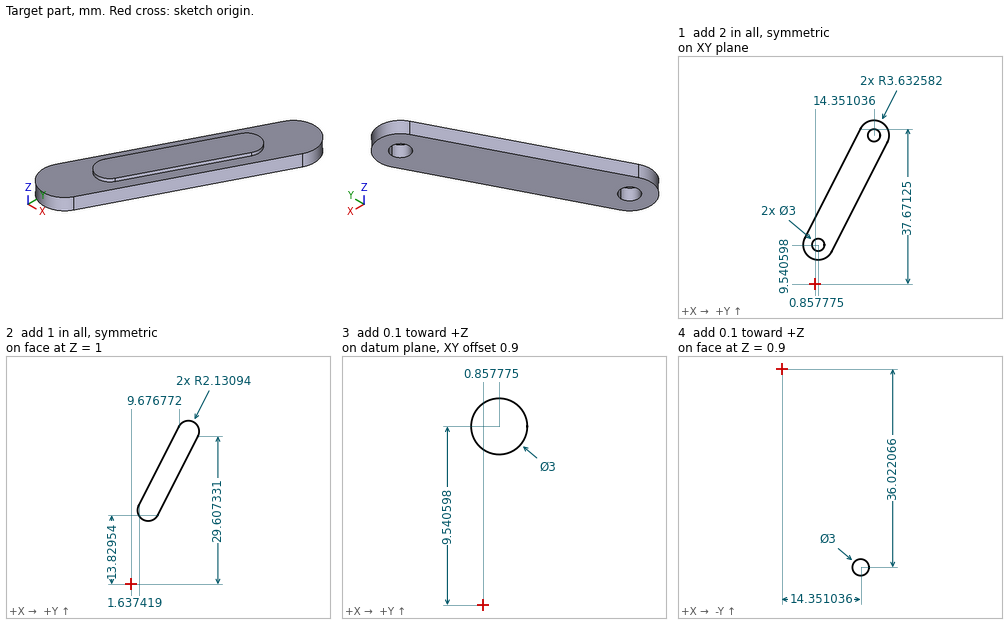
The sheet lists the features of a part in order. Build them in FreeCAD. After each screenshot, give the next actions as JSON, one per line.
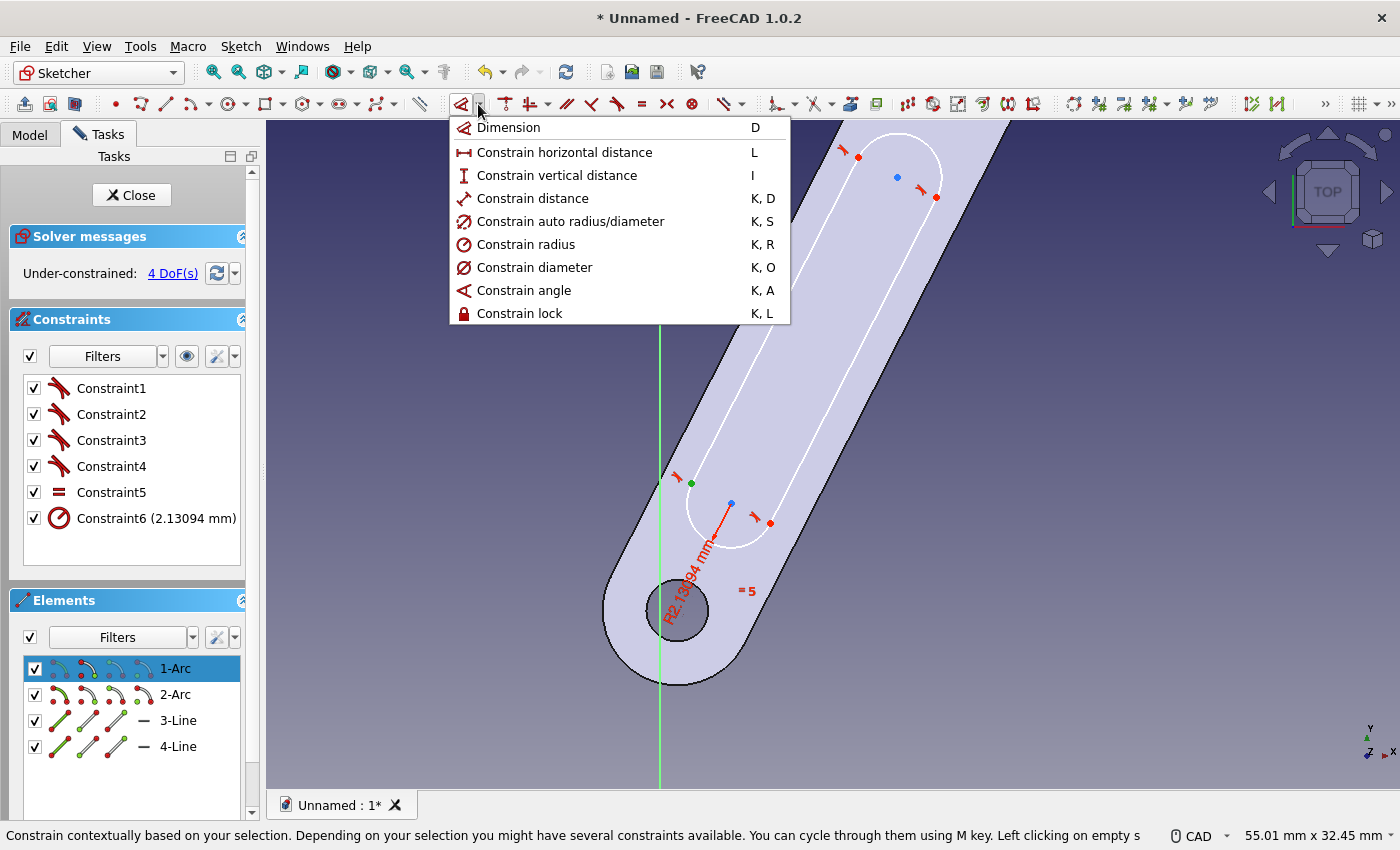
{"action": "left_click", "coordinate": [620, 152]}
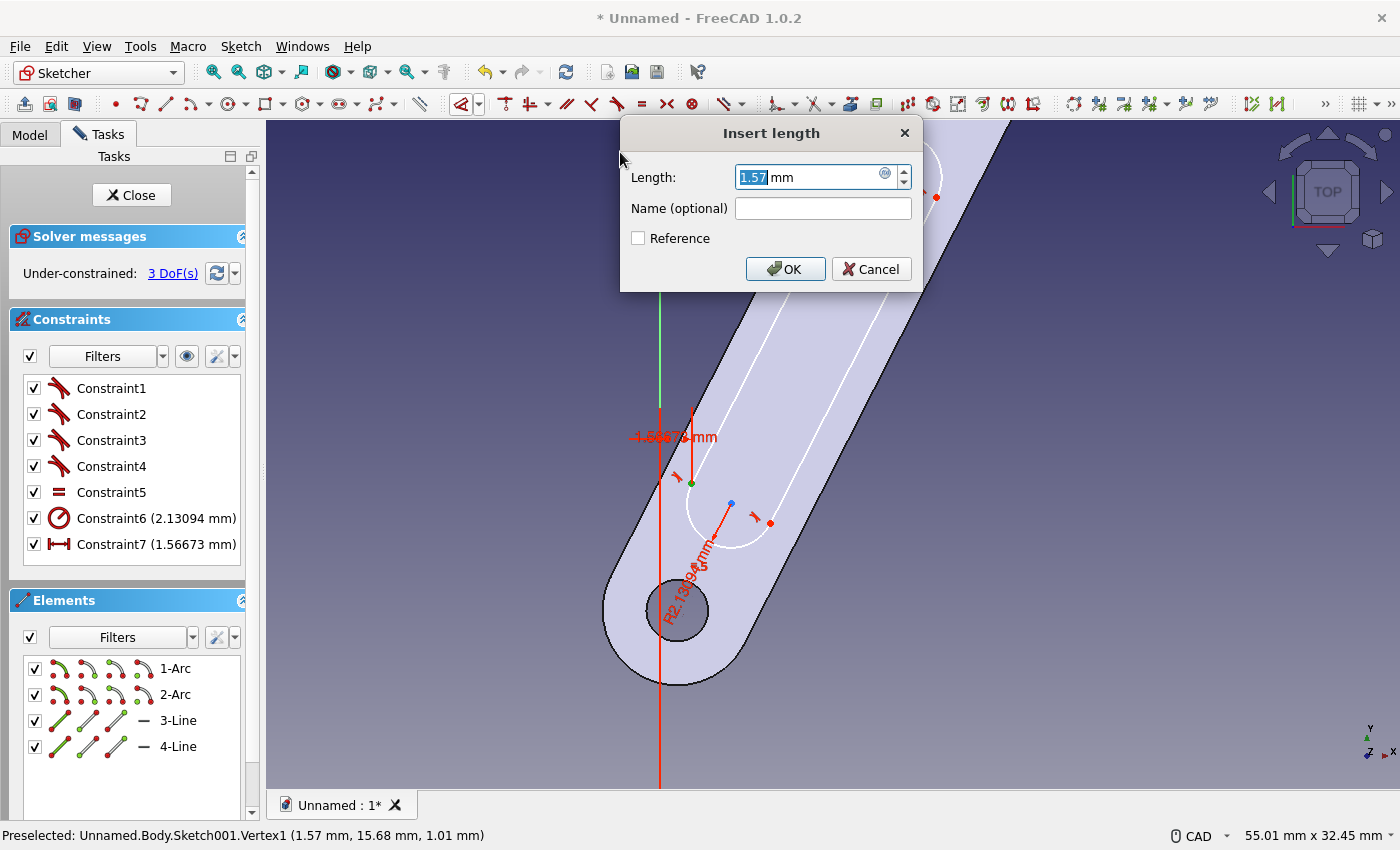
{"action": "type", "text": "1.637419"}
{"action": "key", "text": "Return"}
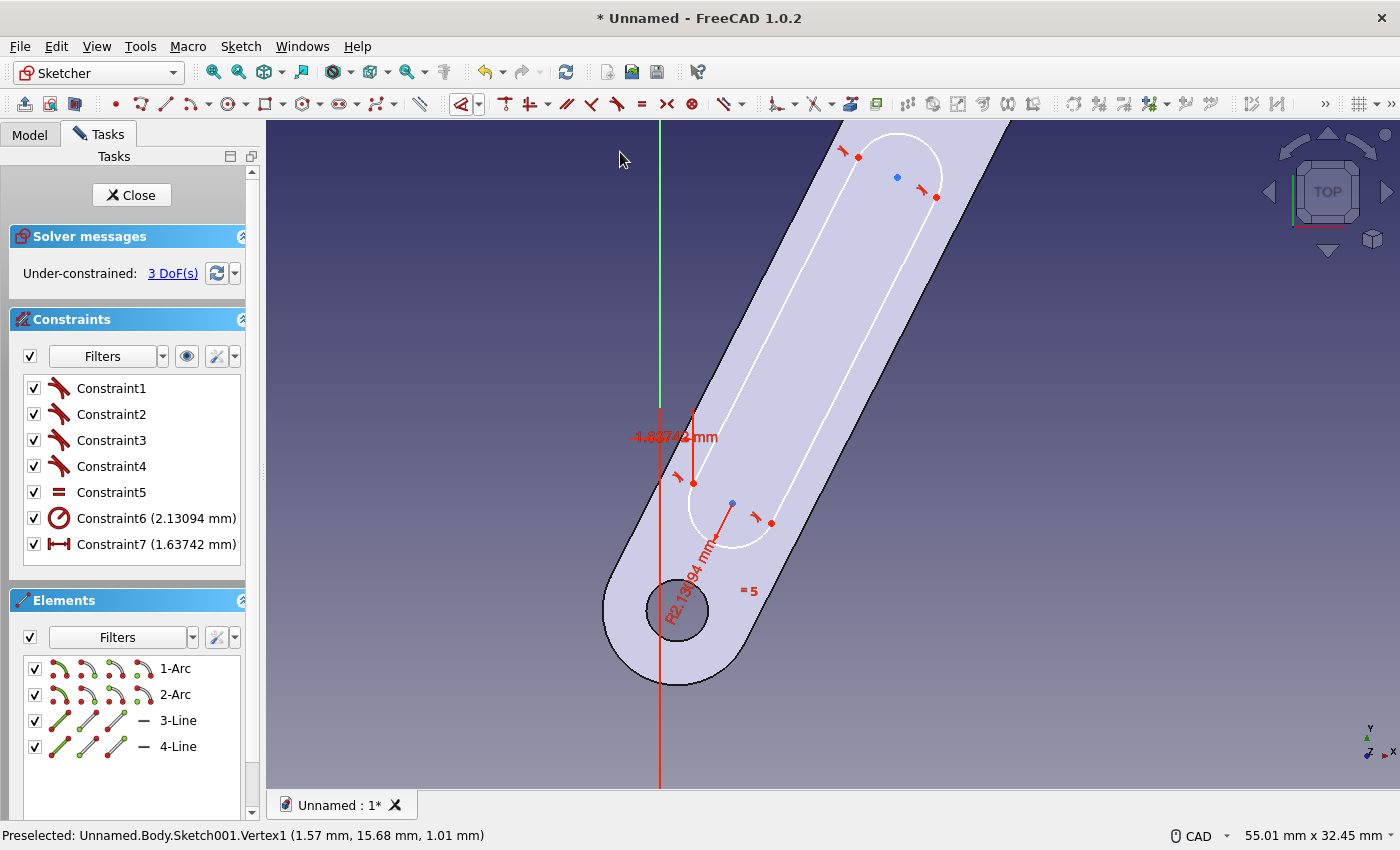
{"action": "left_click", "coordinate": [772, 524]}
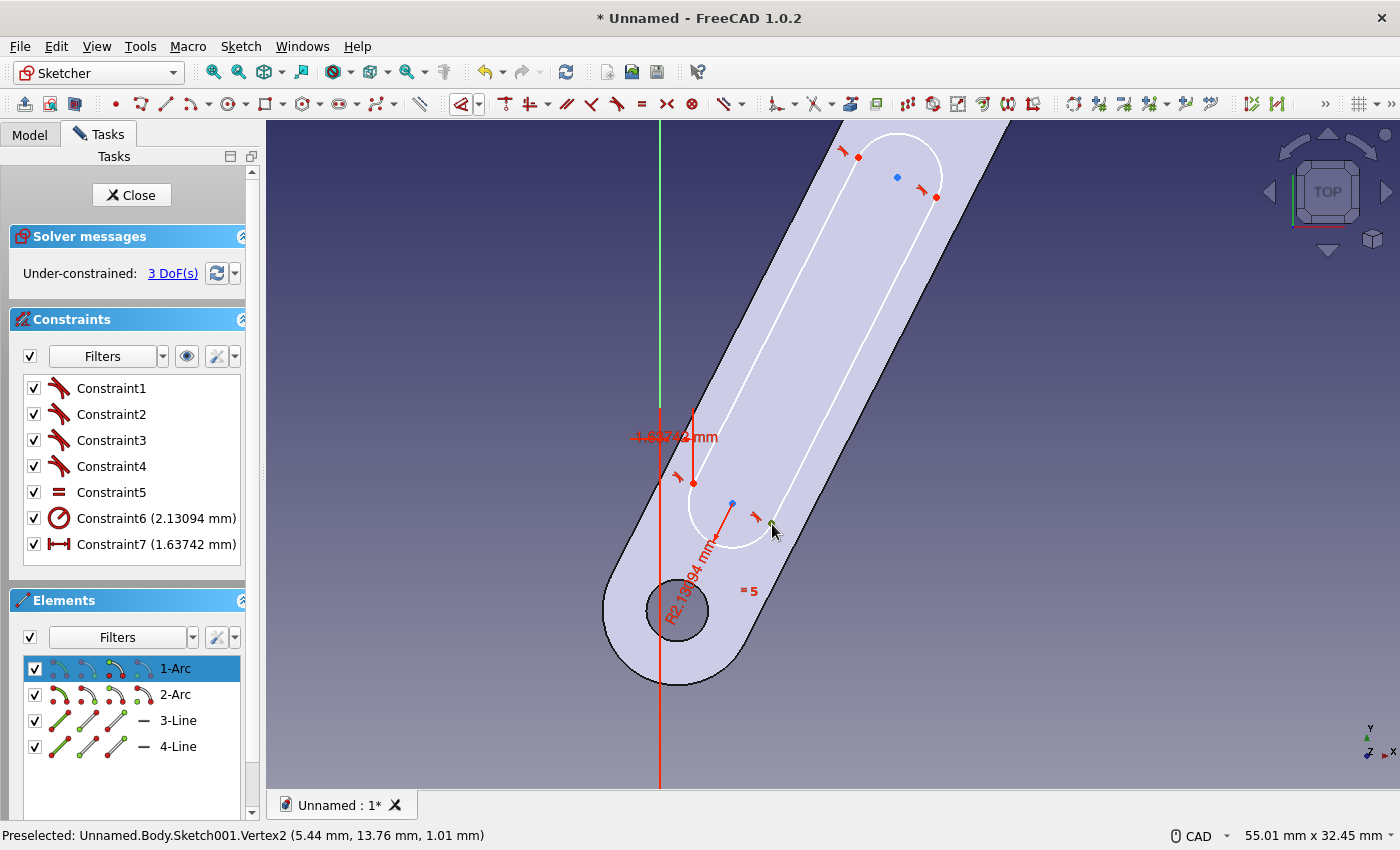
{"action": "key", "text": "i"}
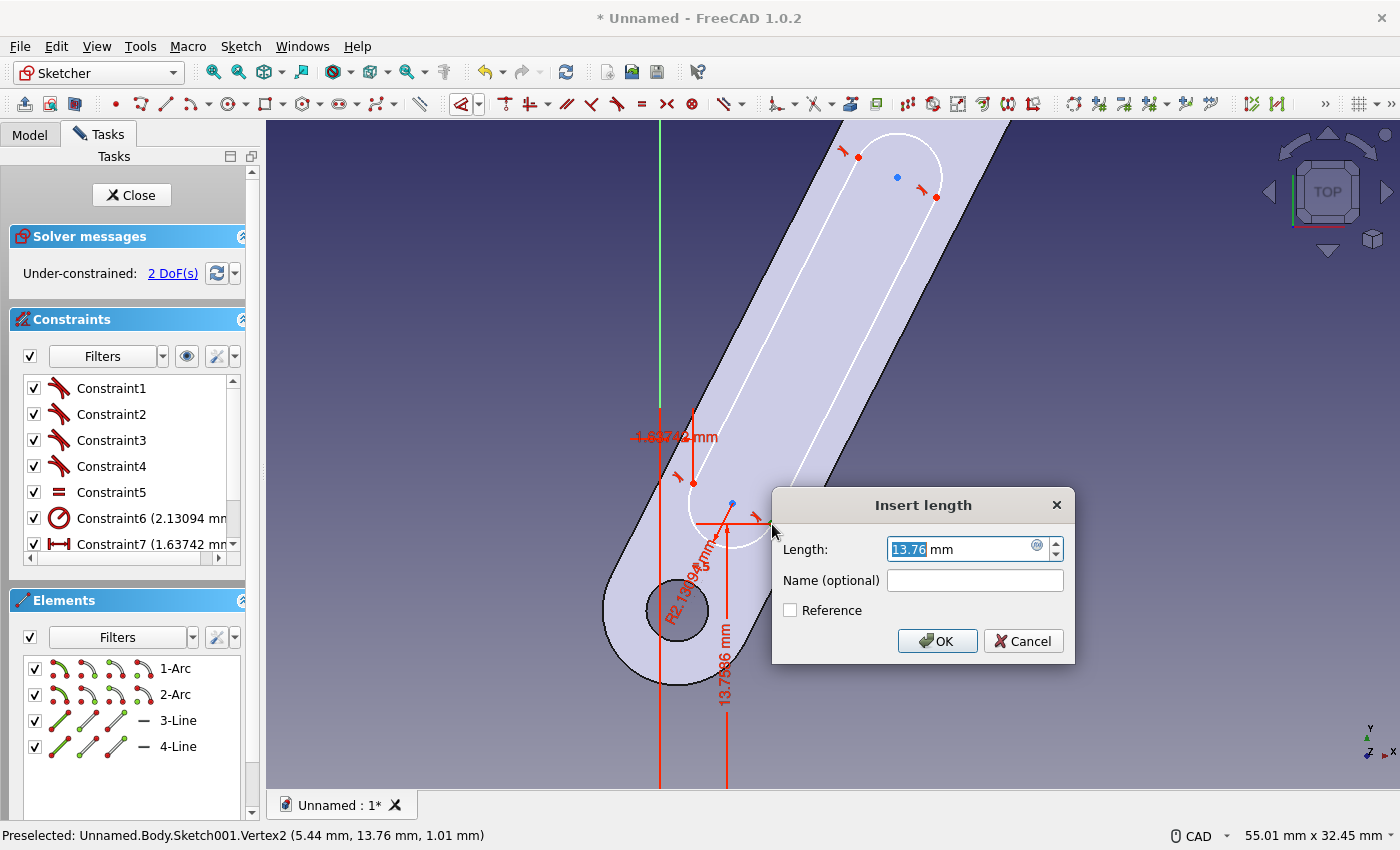
{"action": "type", "text": "13.82954"}
{"action": "key", "text": "Return"}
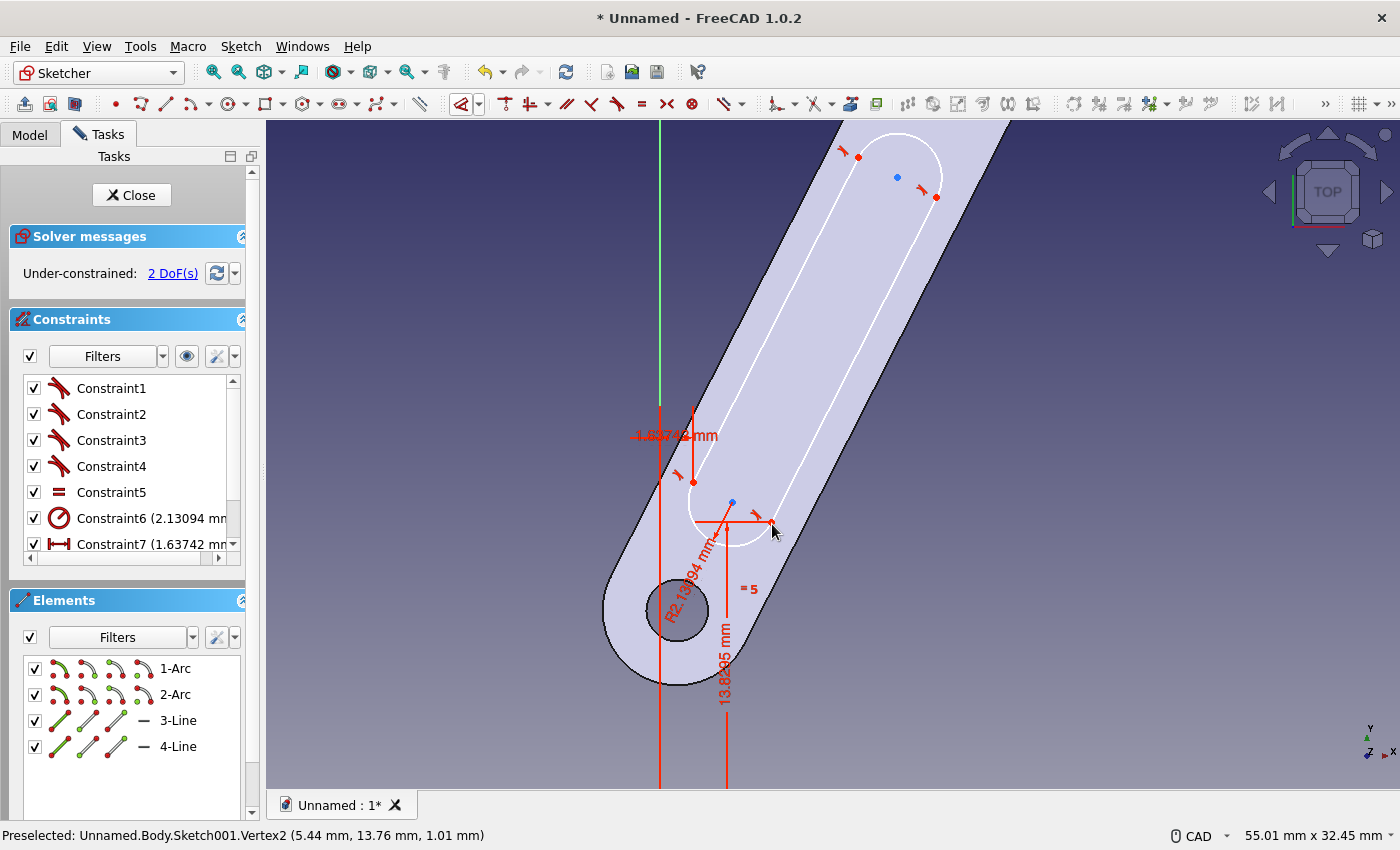
{"action": "left_click", "coordinate": [859, 158]}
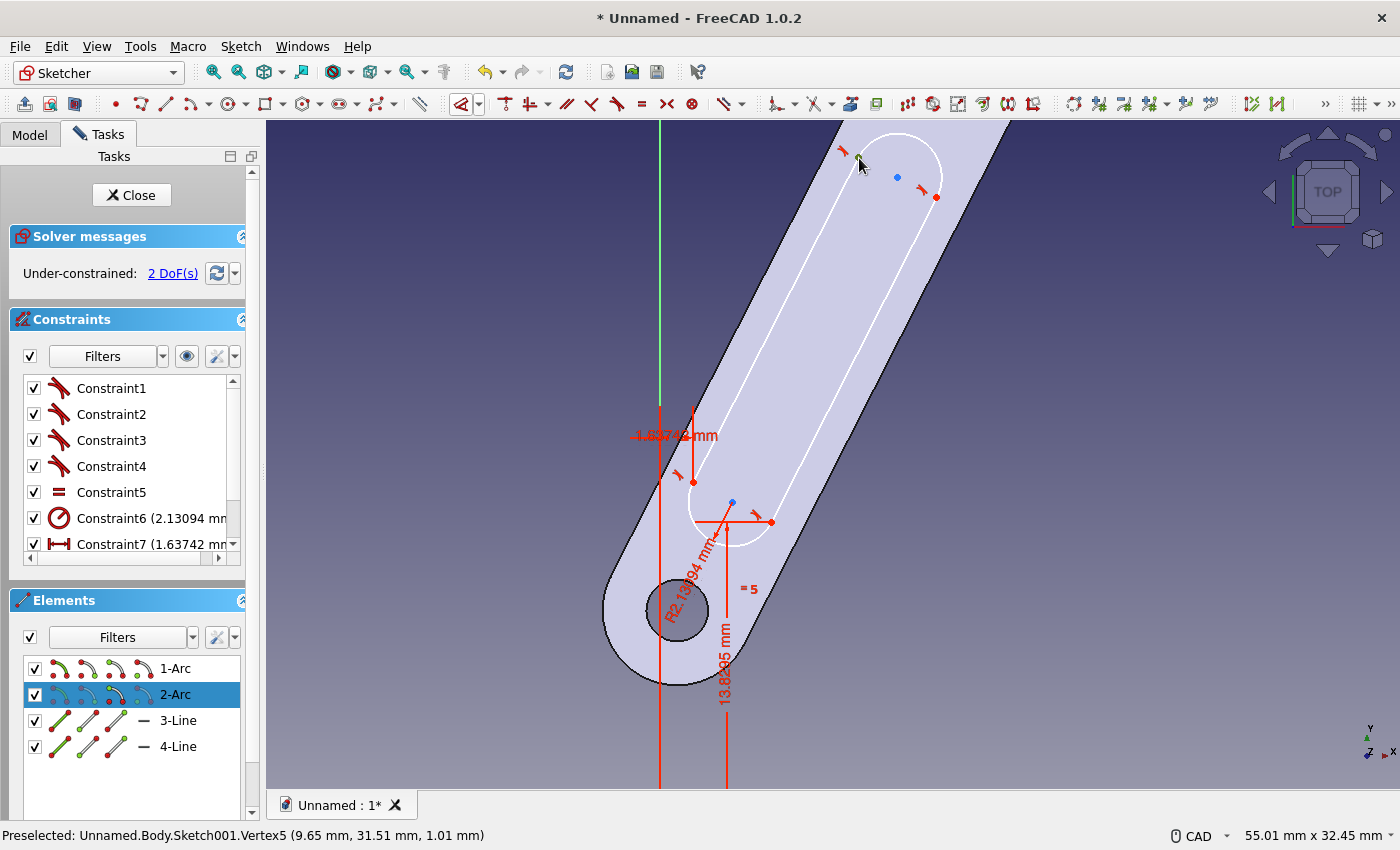
{"action": "left_click", "coordinate": [478, 104]}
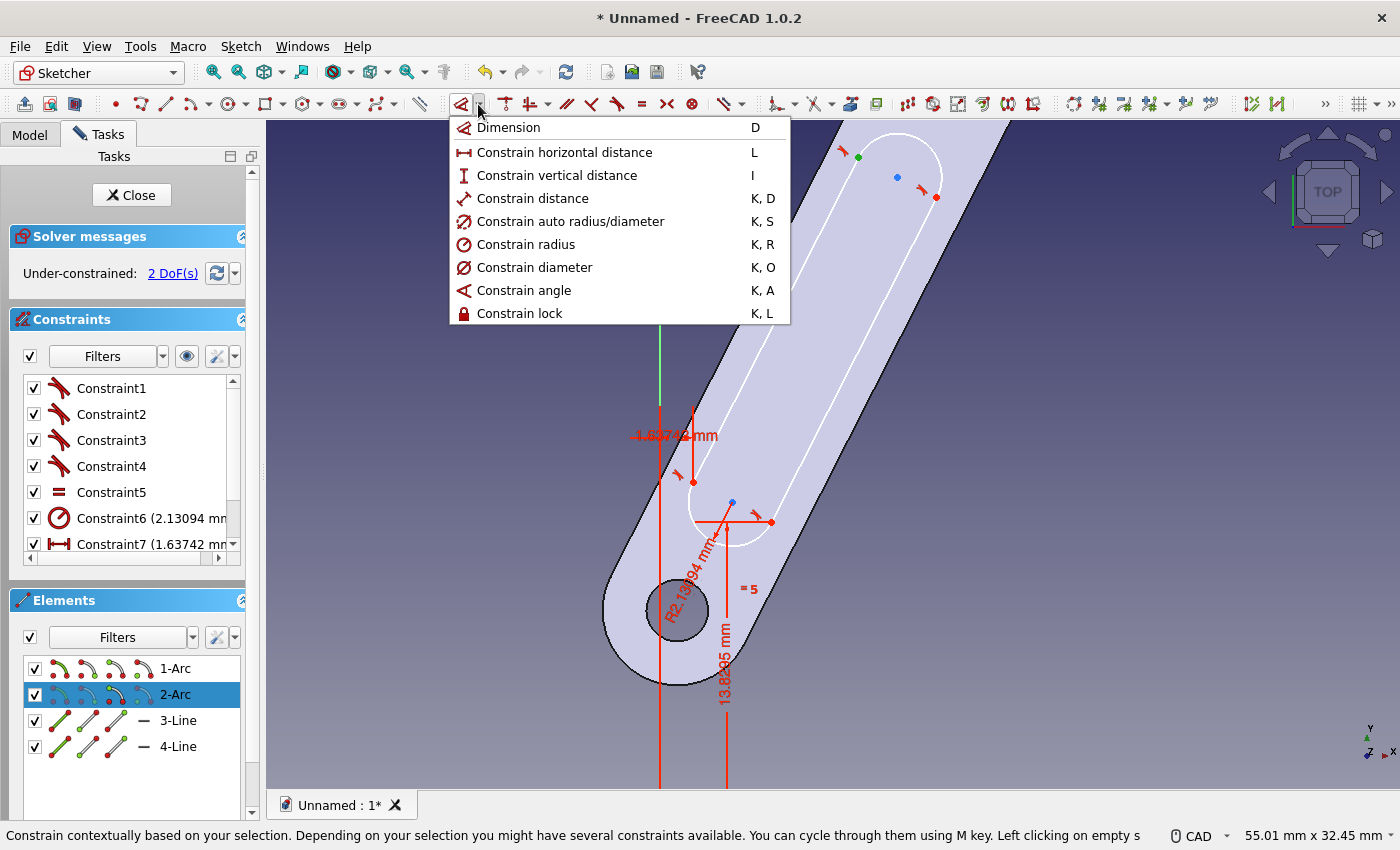
{"action": "left_click", "coordinate": [620, 152]}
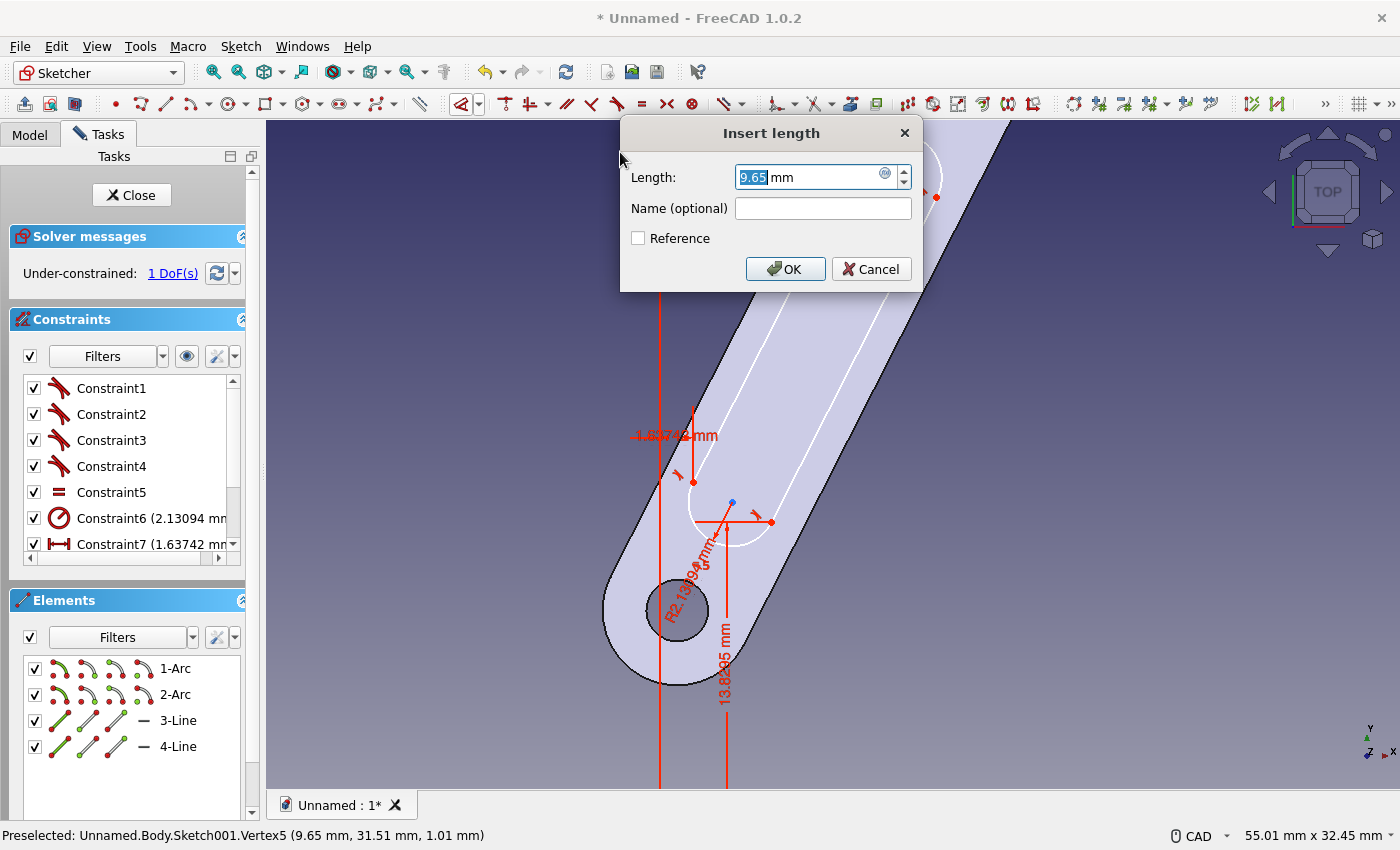
{"action": "type", "text": "9.676772"}
{"action": "key", "text": "Return"}